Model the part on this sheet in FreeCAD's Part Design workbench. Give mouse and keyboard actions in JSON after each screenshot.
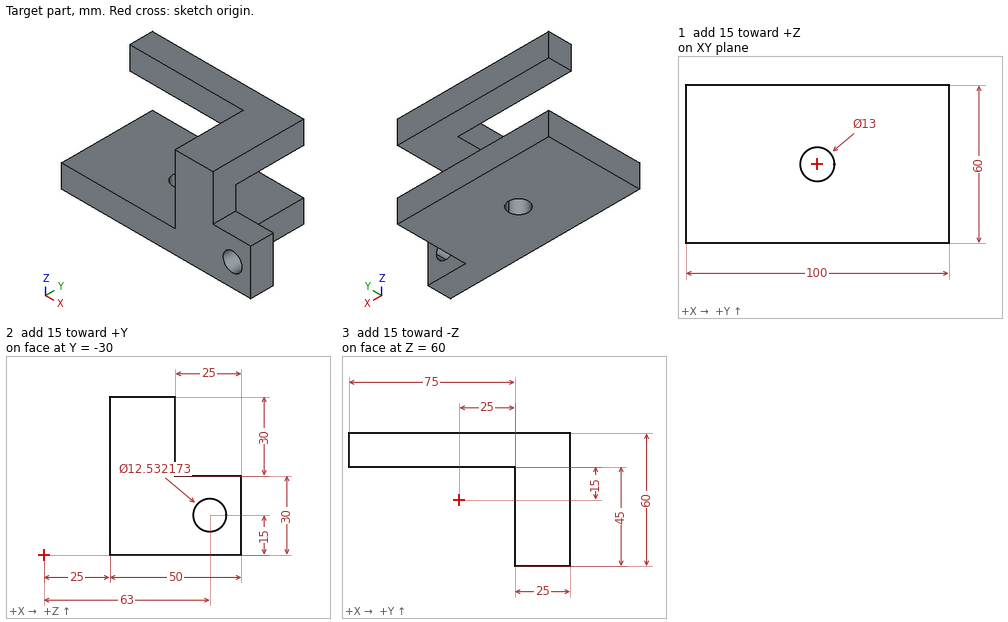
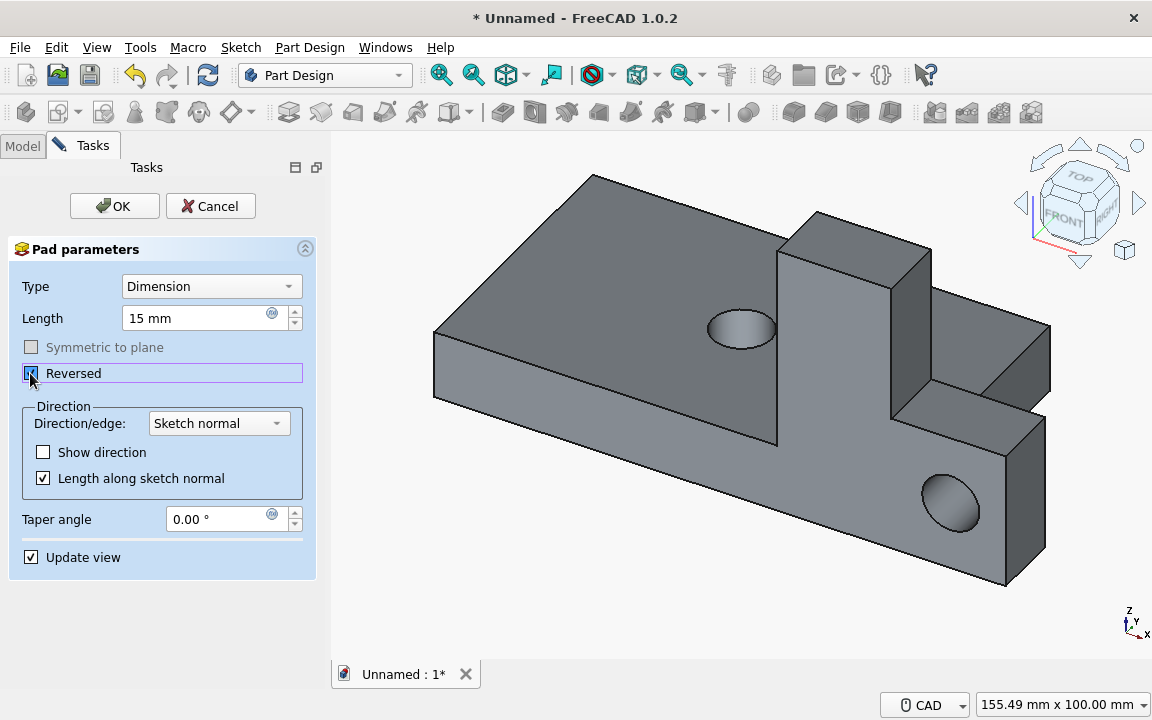
{"action": "left_click", "coordinate": [115, 206]}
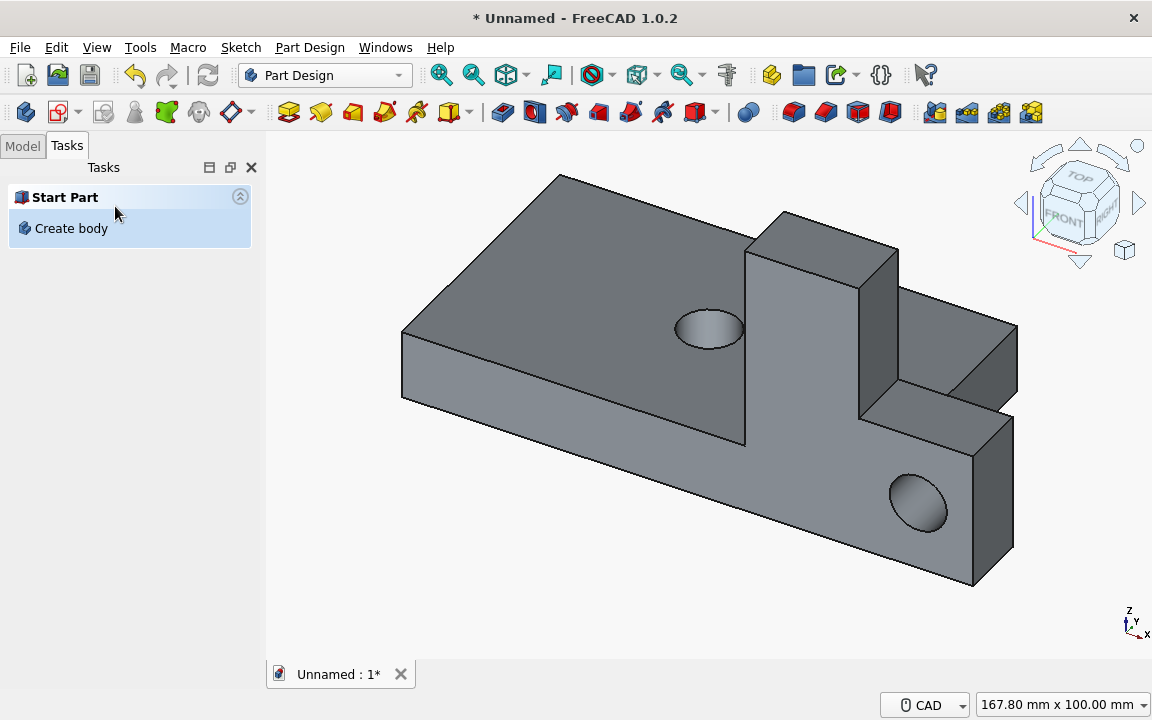
{"action": "left_click", "coordinate": [442, 76]}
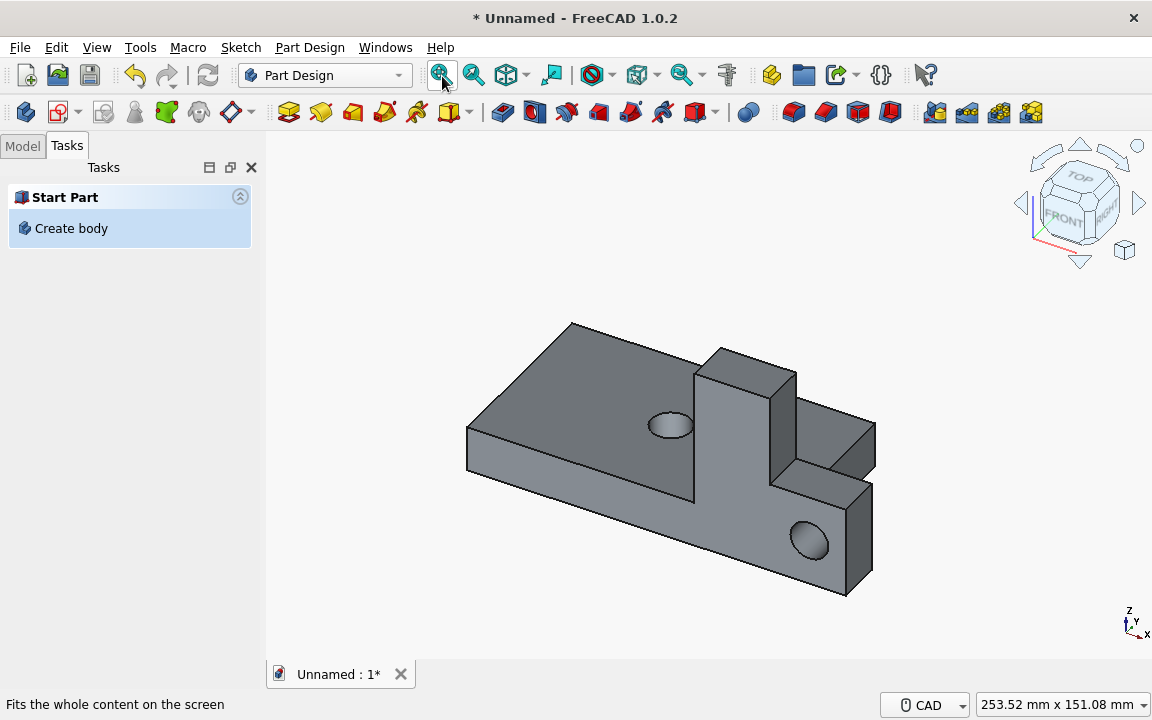
{"action": "left_click", "coordinate": [756, 376]}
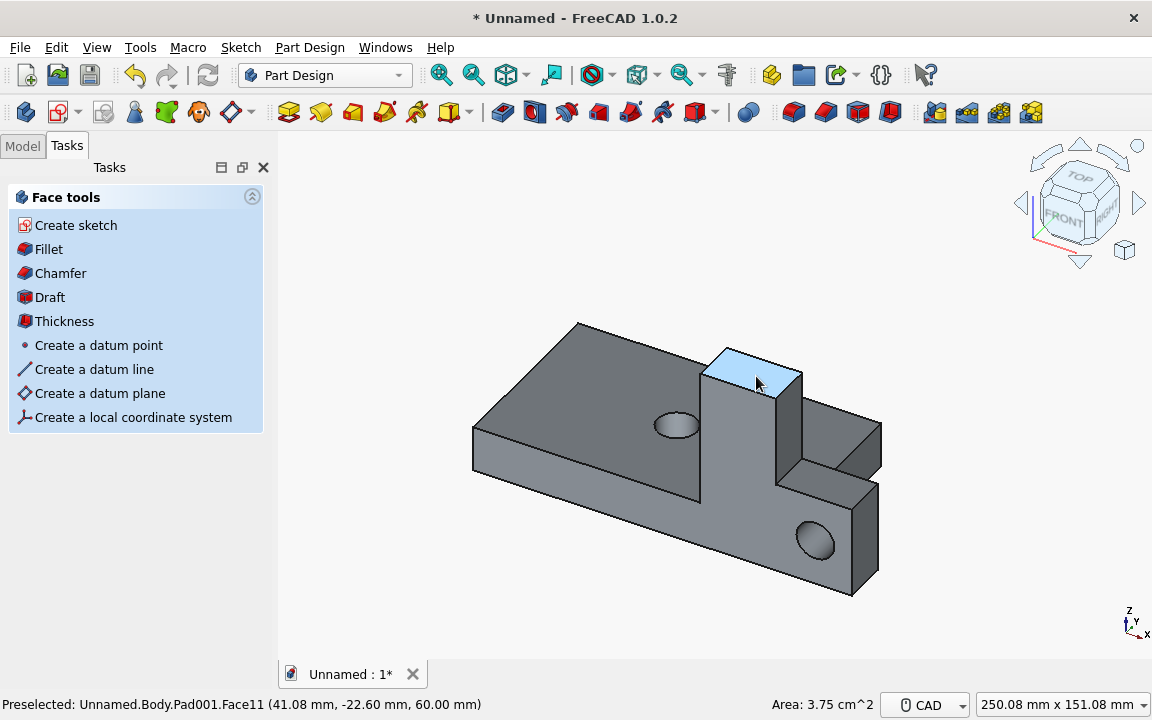
{"action": "left_click", "coordinate": [58, 112]}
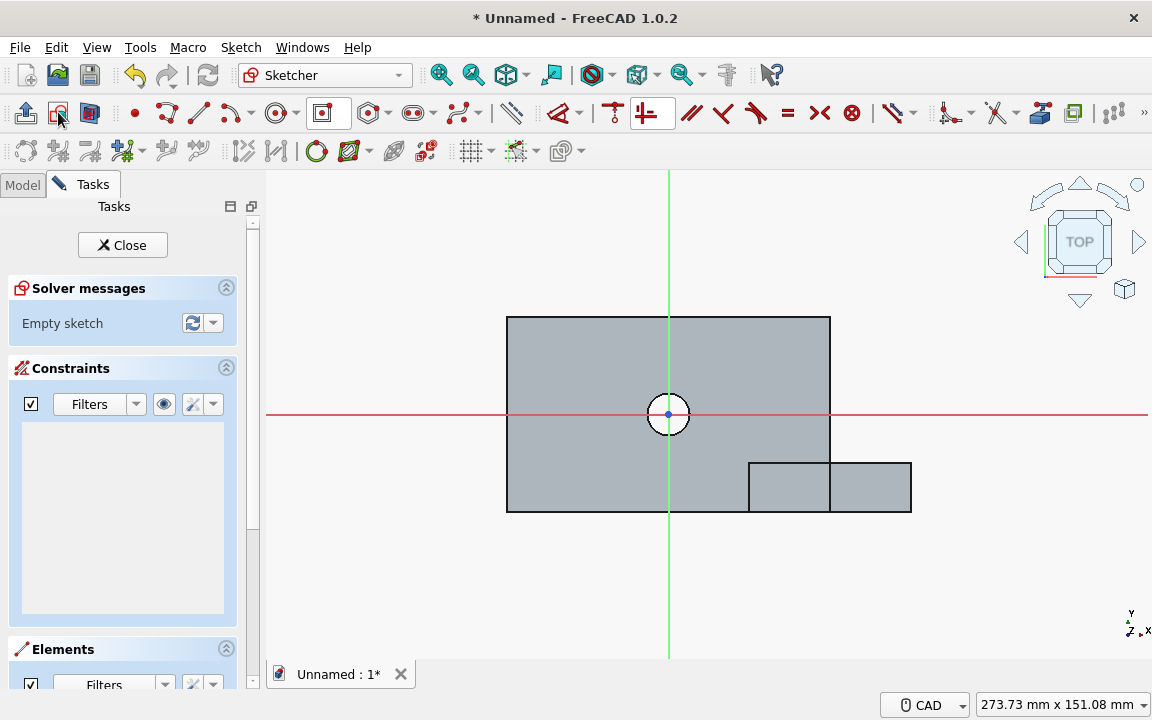
{"action": "scroll", "coordinate": [726, 414], "scroll_direction": "up", "scroll_amount": 2}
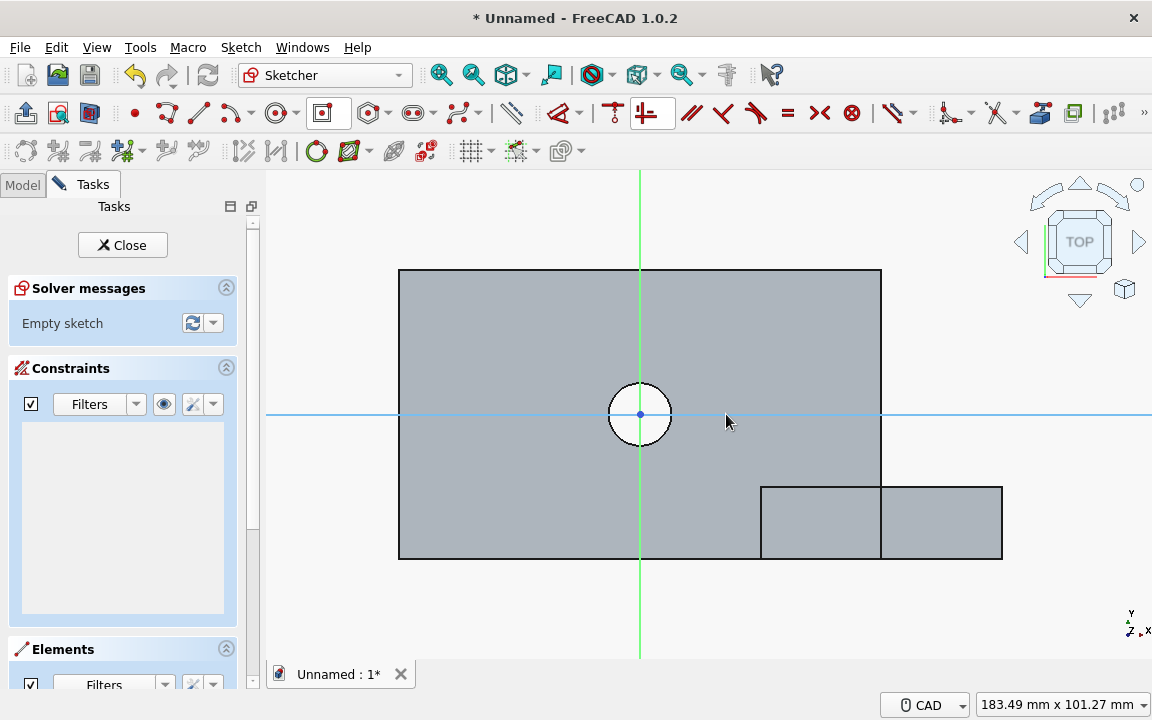
{"action": "key", "text": "g m"}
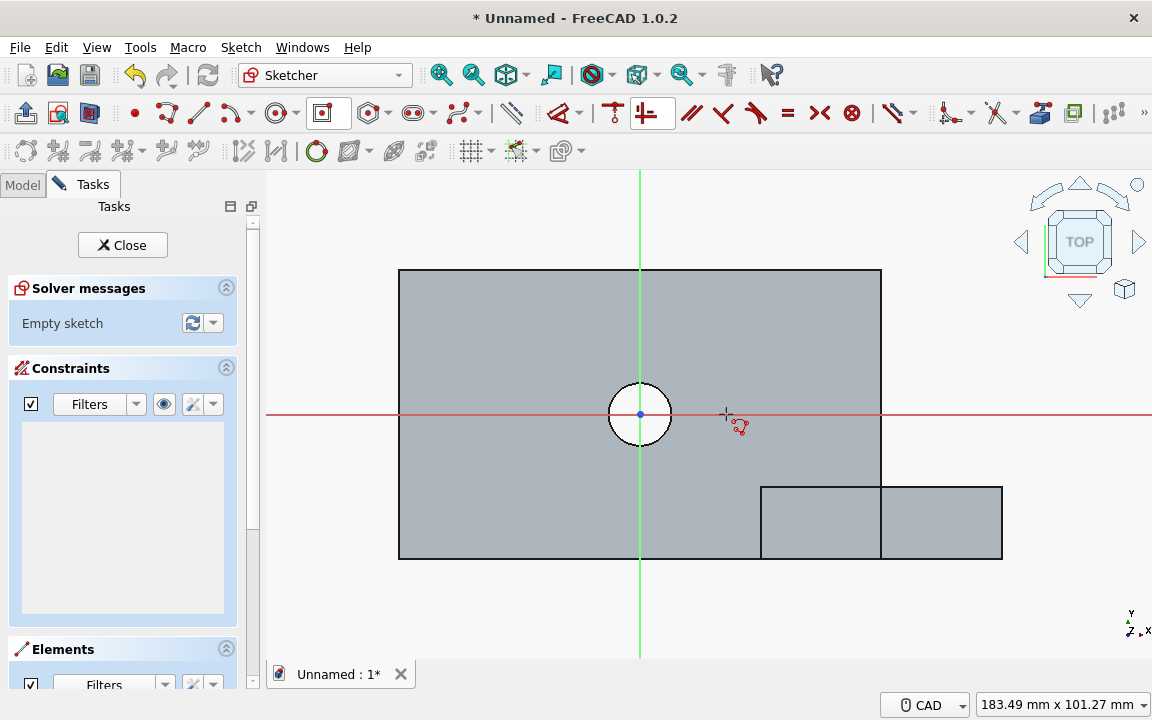
{"action": "left_click", "coordinate": [761, 342]}
{"action": "left_click", "coordinate": [761, 559]}
{"action": "left_click", "coordinate": [881, 559]}
{"action": "left_click", "coordinate": [881, 270]}
{"action": "left_click", "coordinate": [399, 270]}
{"action": "left_click", "coordinate": [399, 342]}
{"action": "left_click", "coordinate": [761, 343]}
{"action": "key", "text": "Escape"}
{"action": "key", "text": "Escape"}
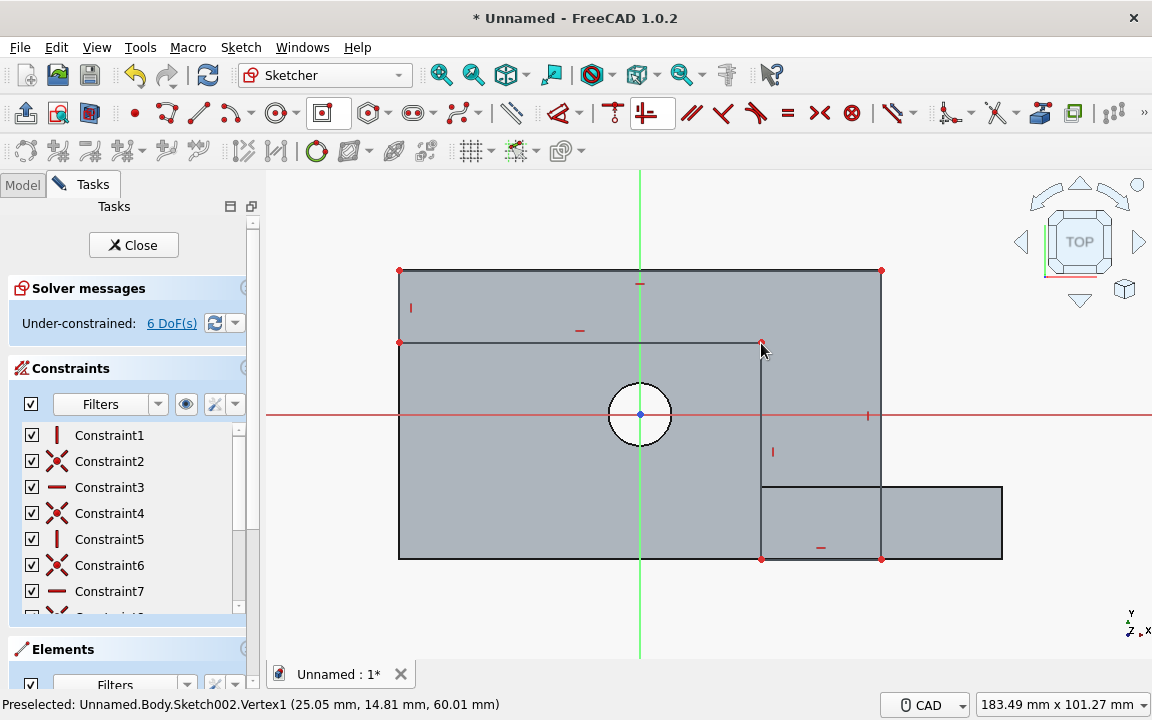
{"action": "left_click", "coordinate": [558, 114]}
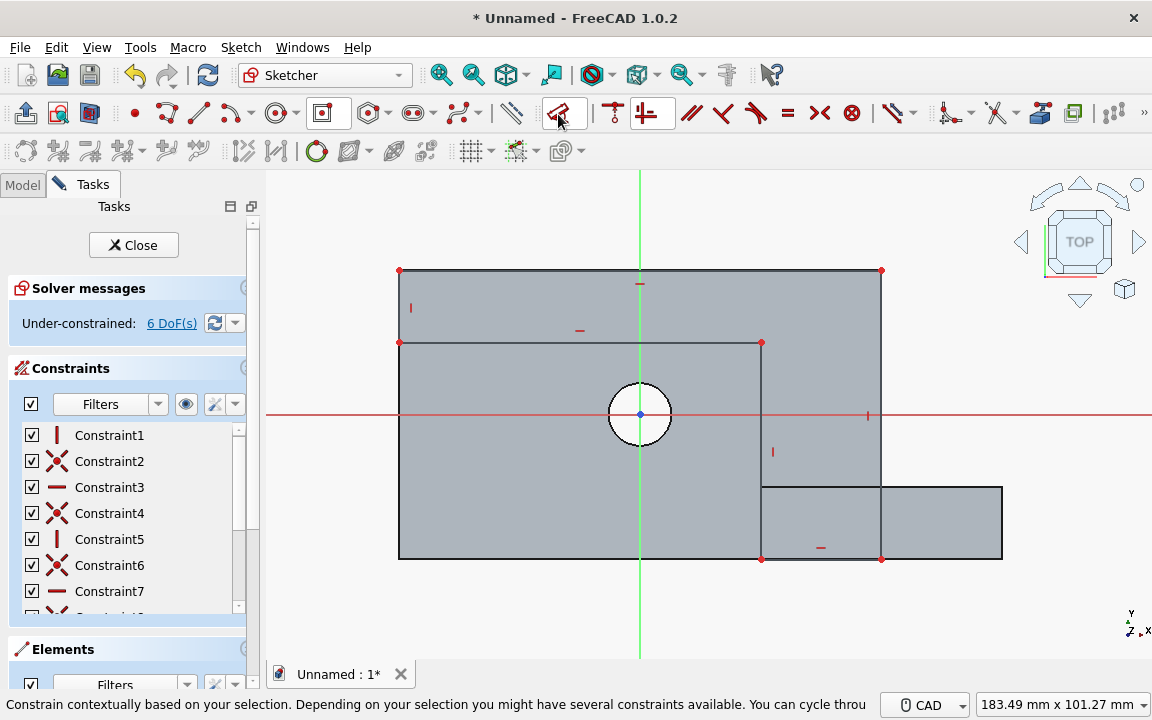
{"action": "left_click", "coordinate": [761, 495]}
{"action": "left_click", "coordinate": [795, 452]}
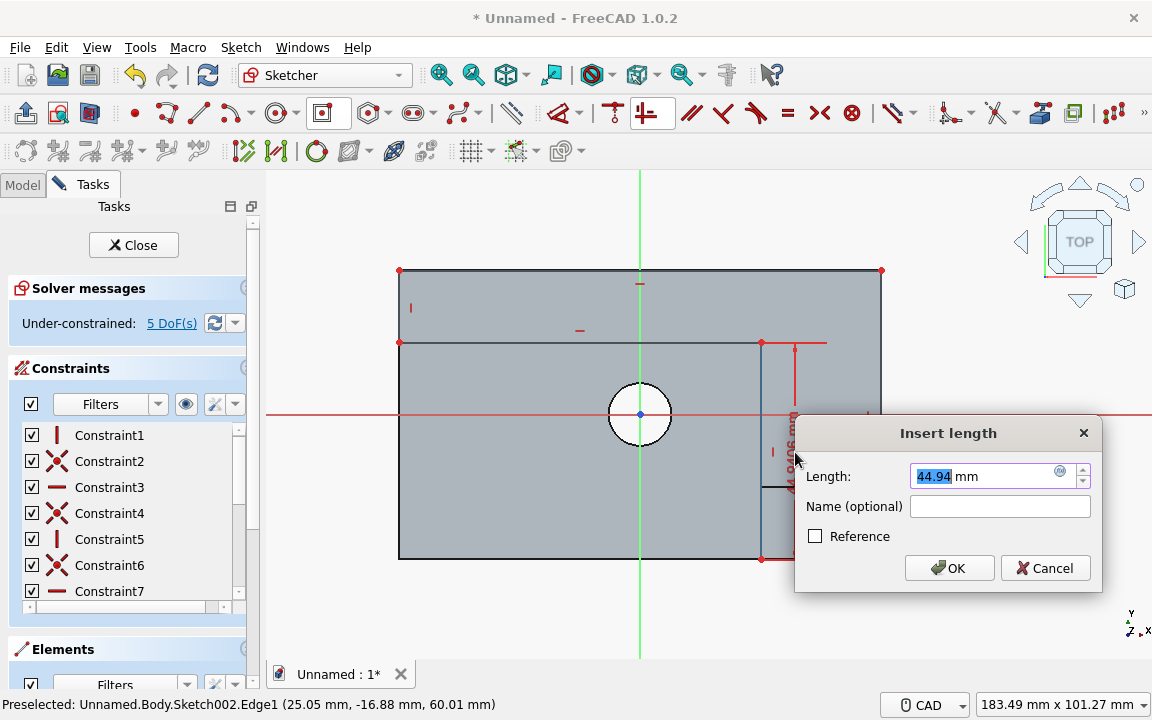
{"action": "type", "text": "45"}
{"action": "key", "text": "Return"}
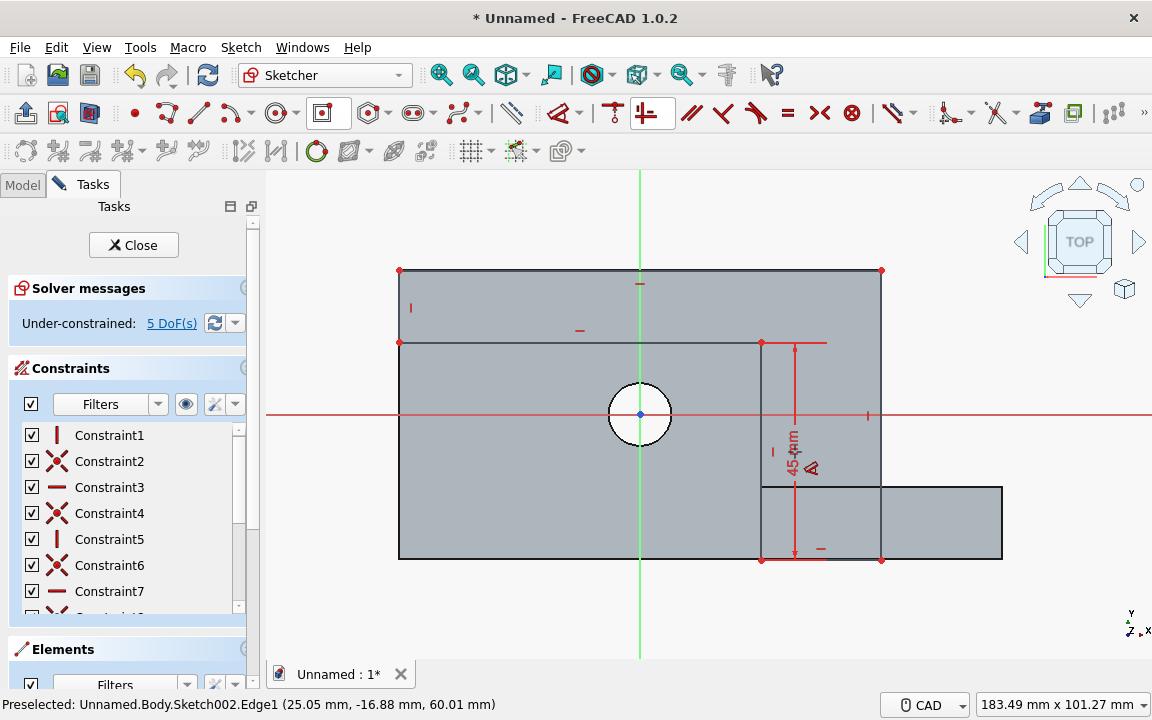
{"action": "left_click", "coordinate": [797, 560]}
{"action": "left_click", "coordinate": [821, 594]}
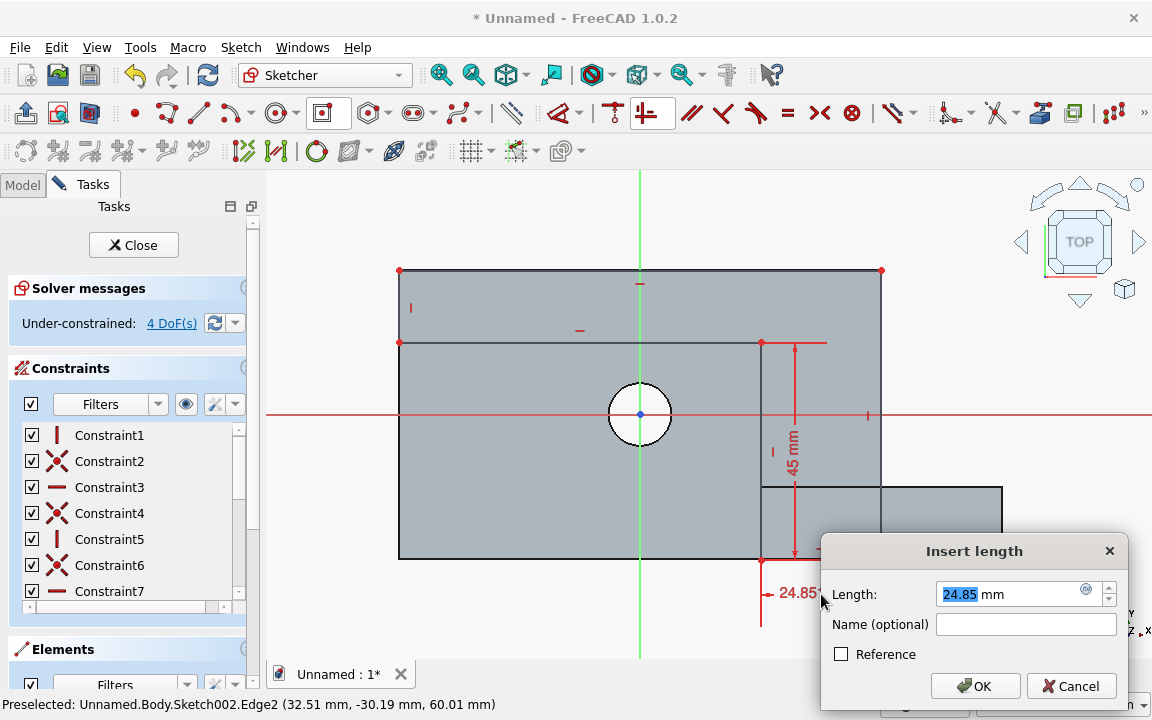
{"action": "type", "text": "25"}
{"action": "key", "text": "Return"}